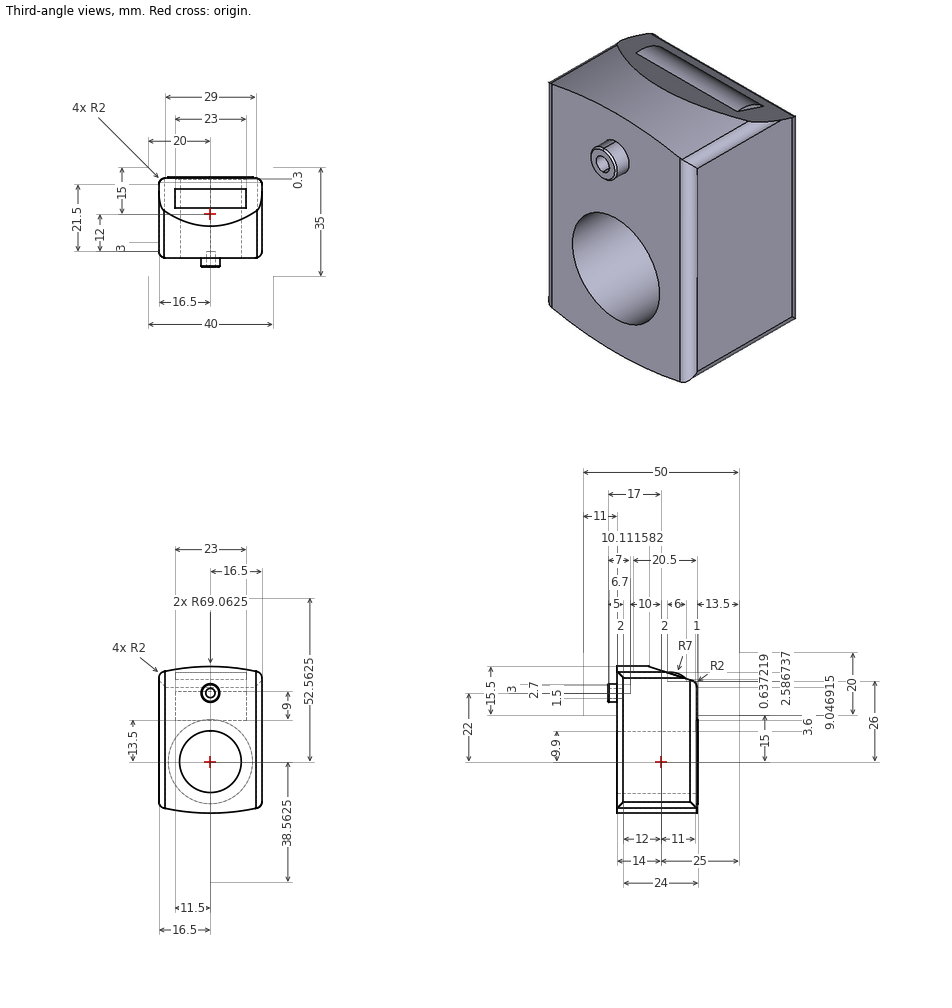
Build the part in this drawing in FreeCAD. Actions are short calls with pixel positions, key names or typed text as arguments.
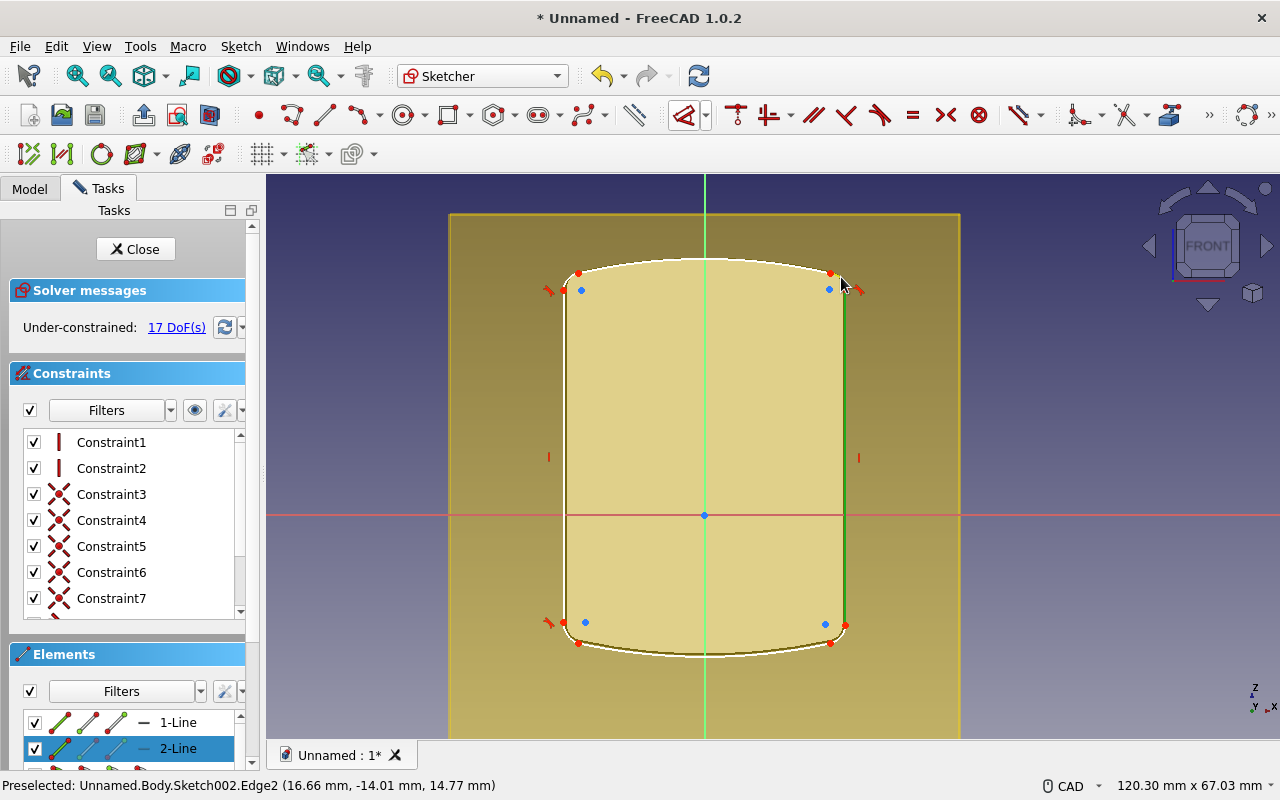
scroll(837, 640, up, 4)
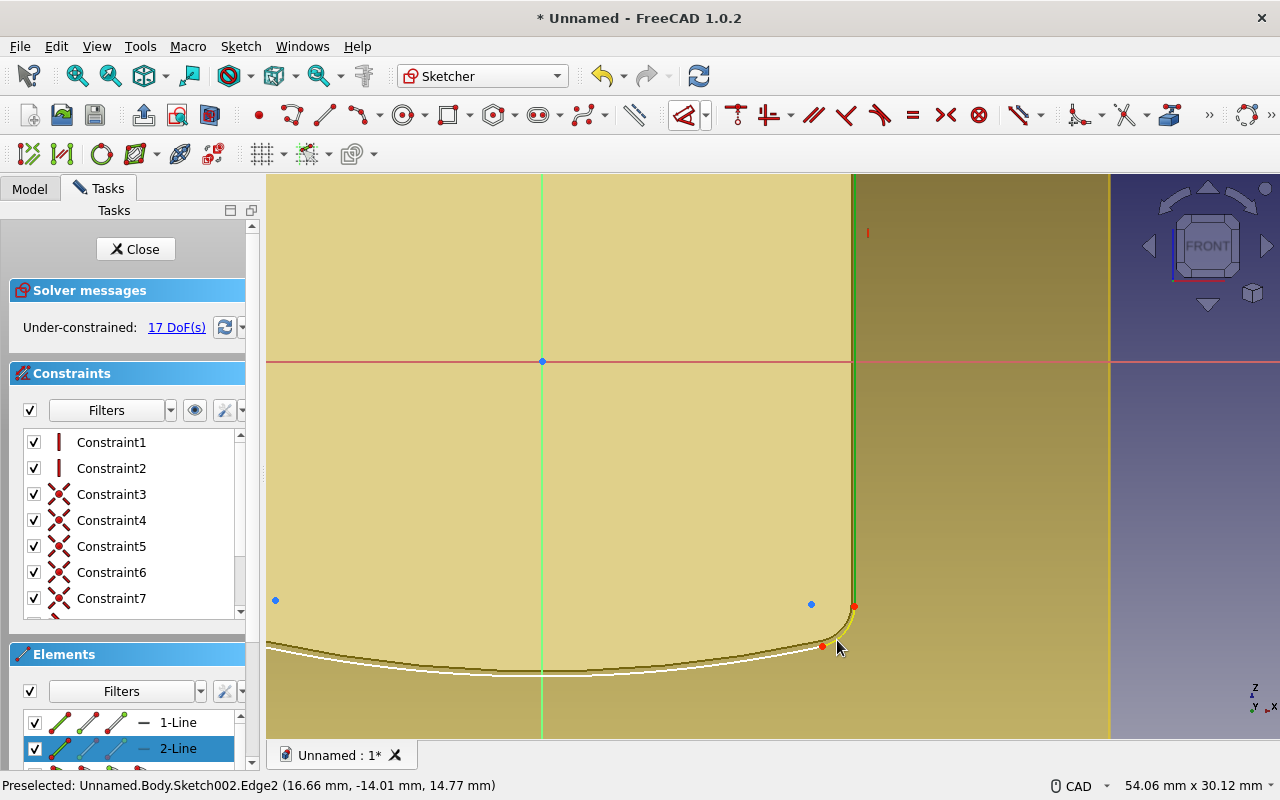
click(837, 639)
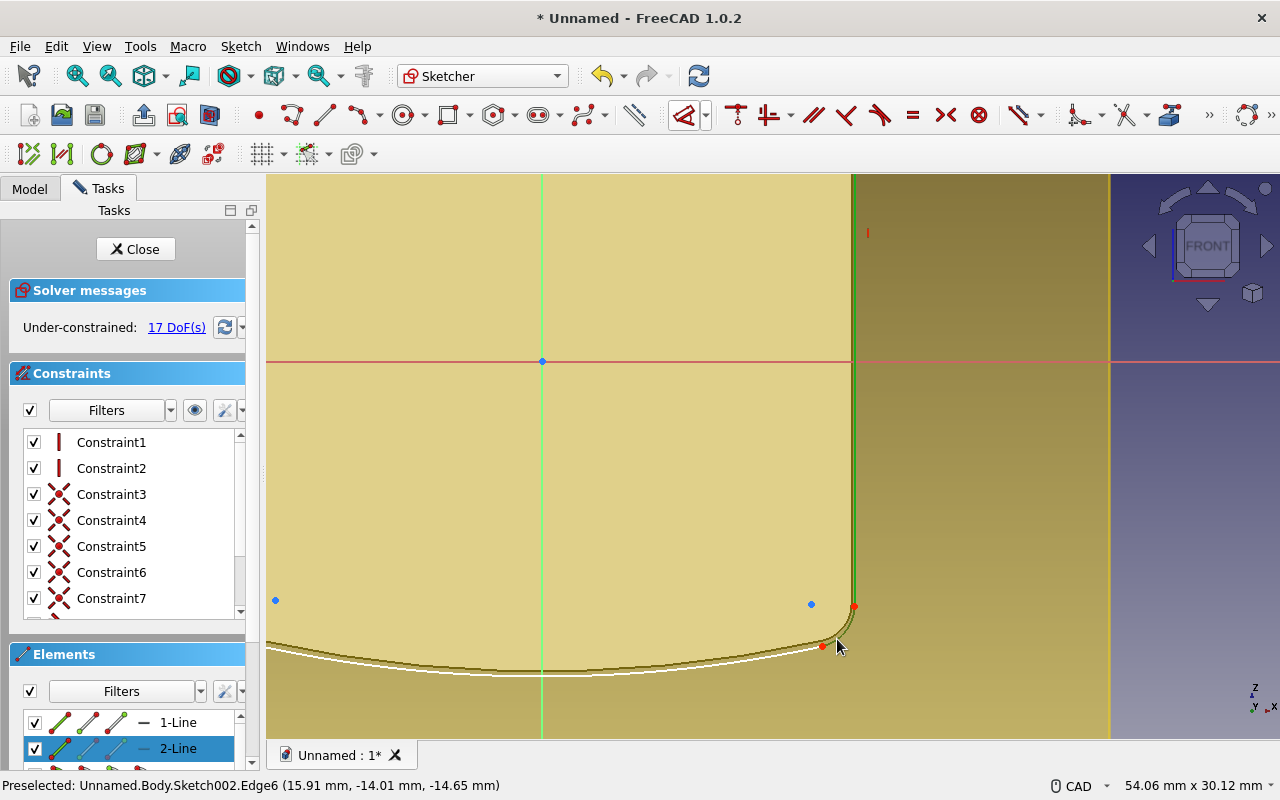
click(880, 116)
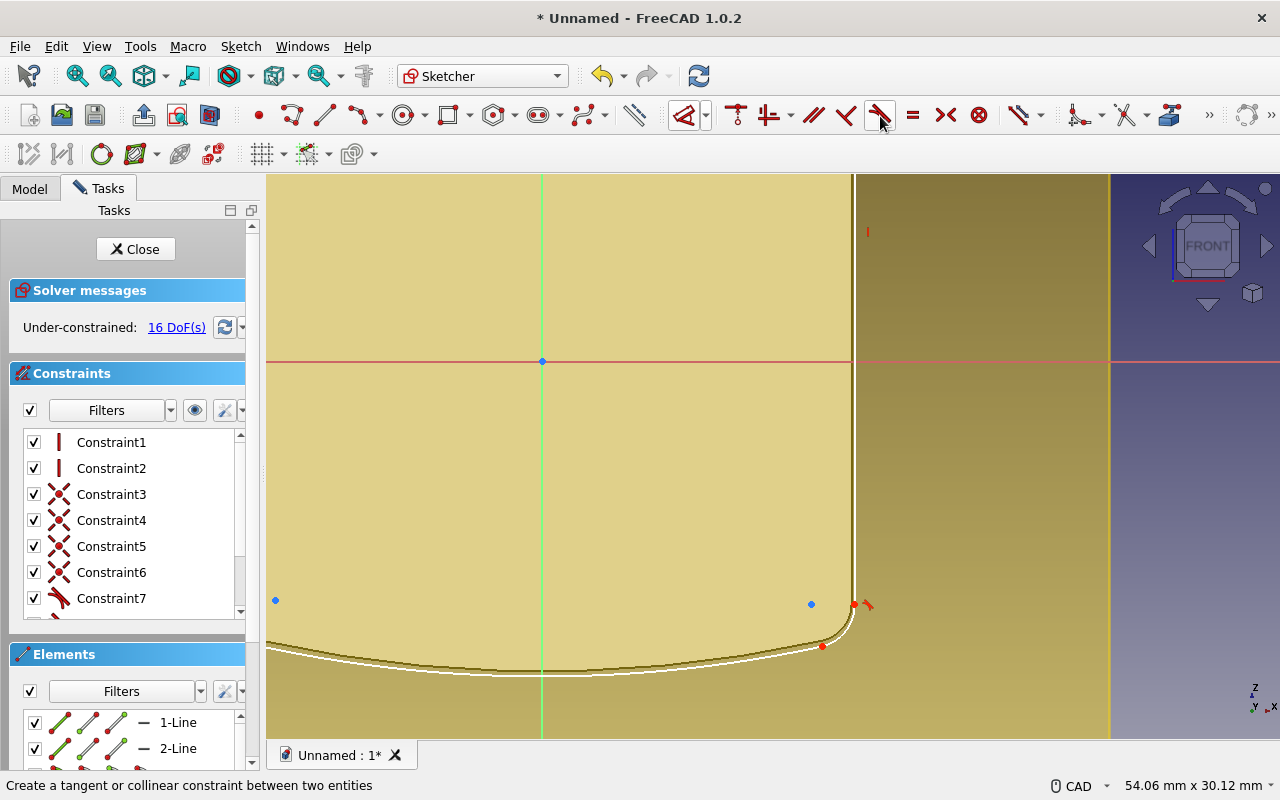
scroll(837, 641, down, 4)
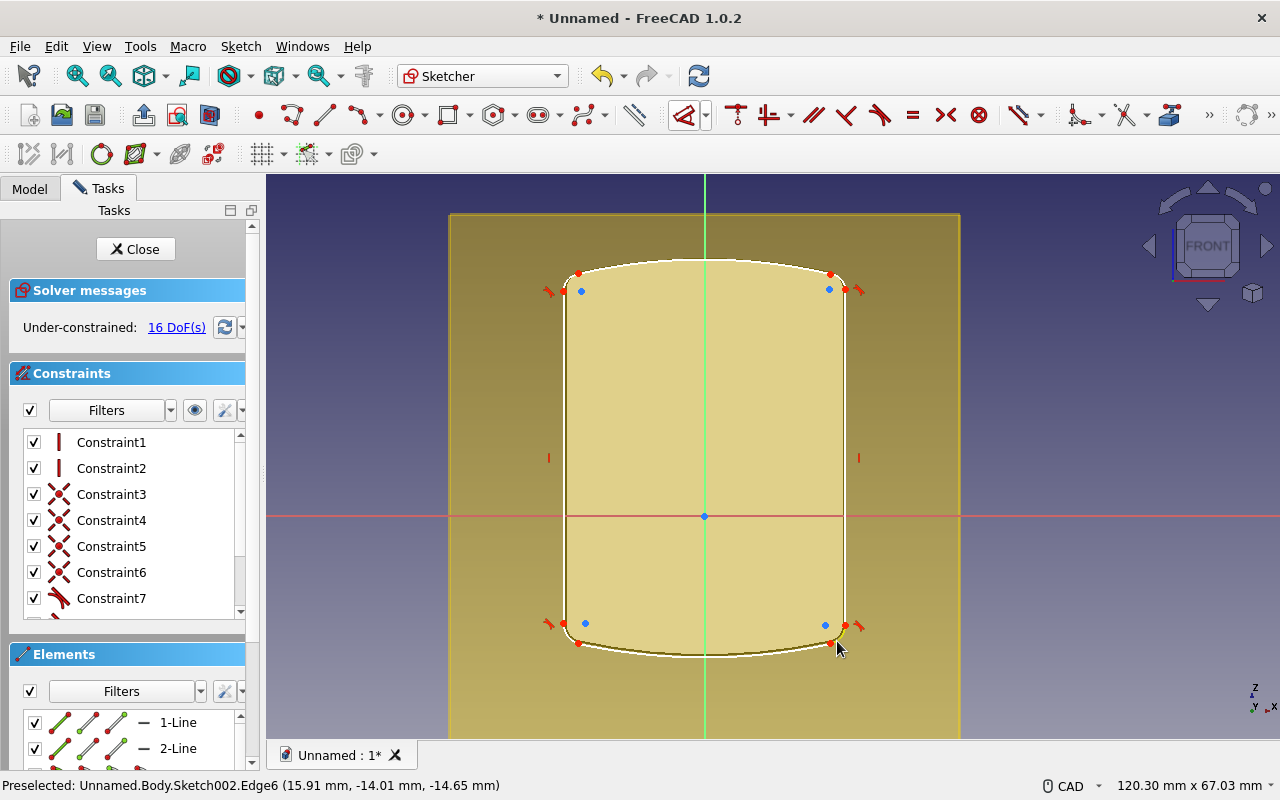
scroll(572, 277, up, 4)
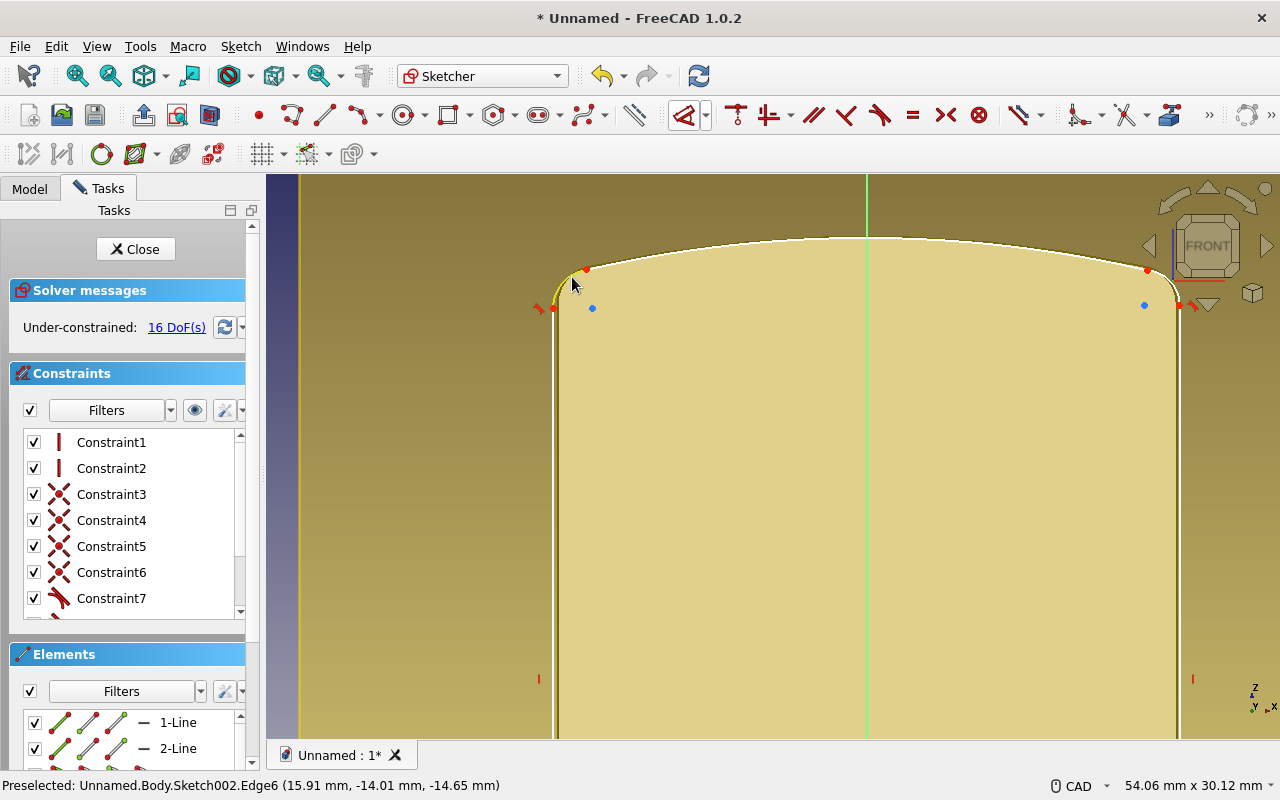
click(571, 276)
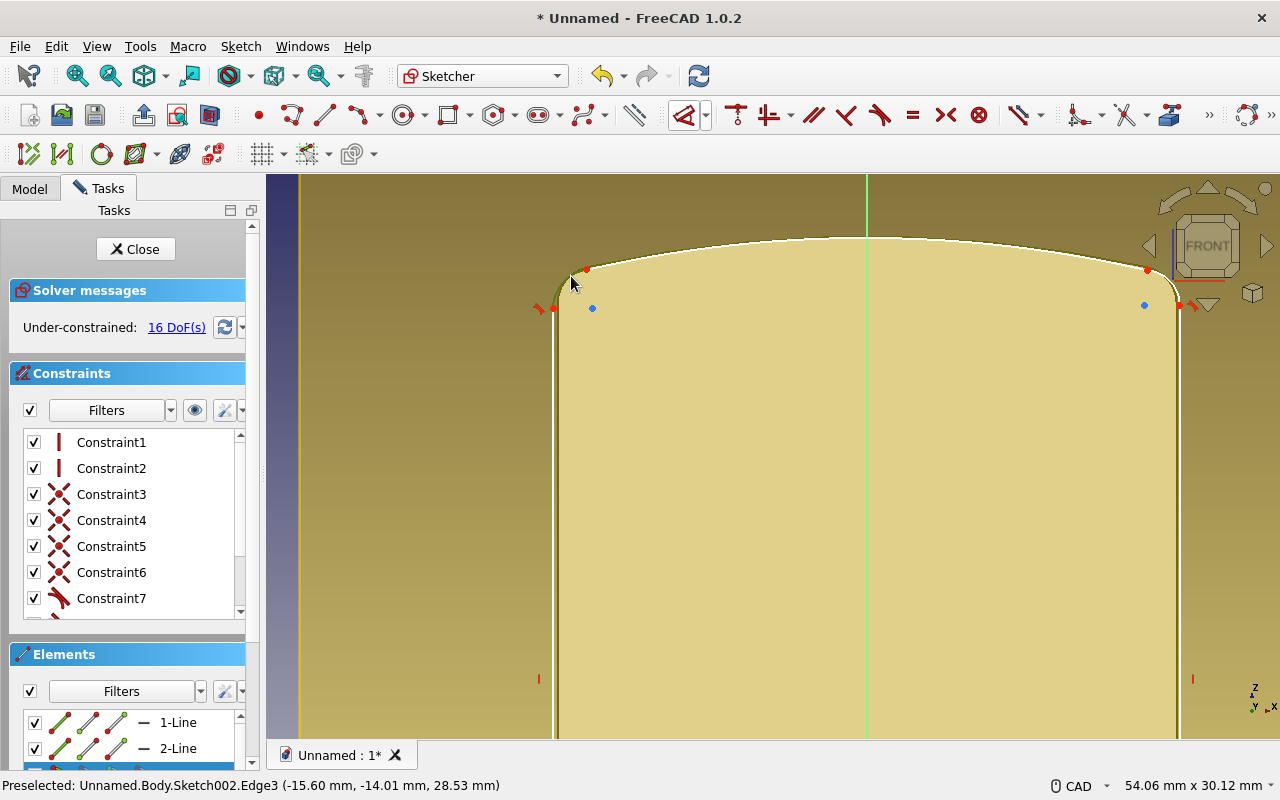
click(980, 243)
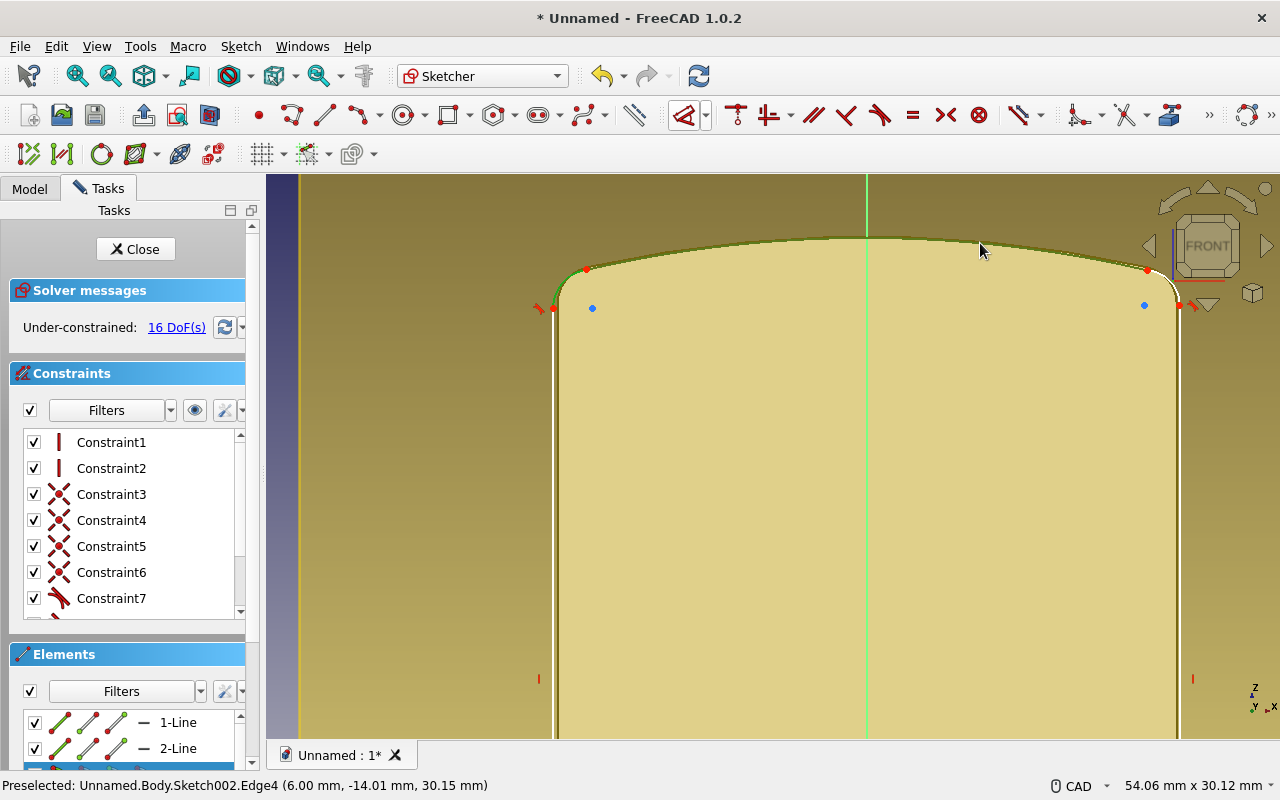
click(880, 116)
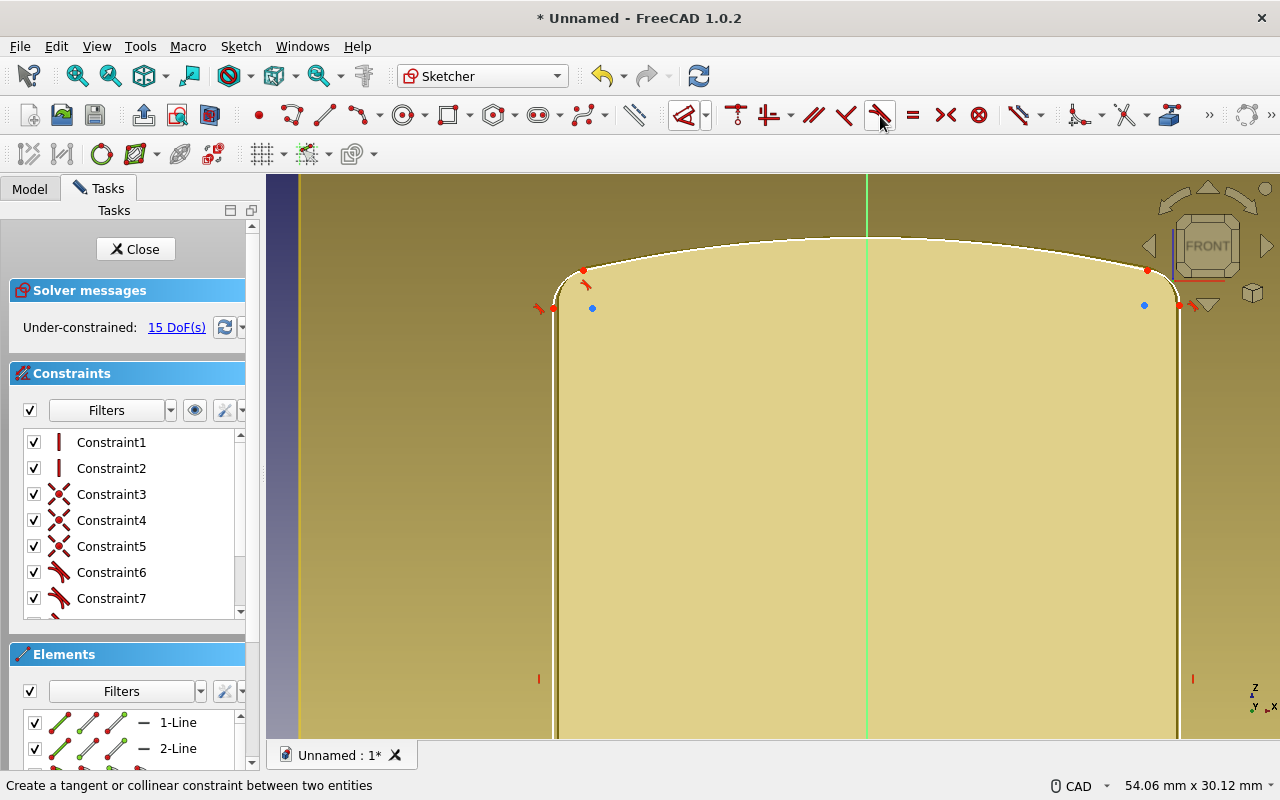
click(979, 243)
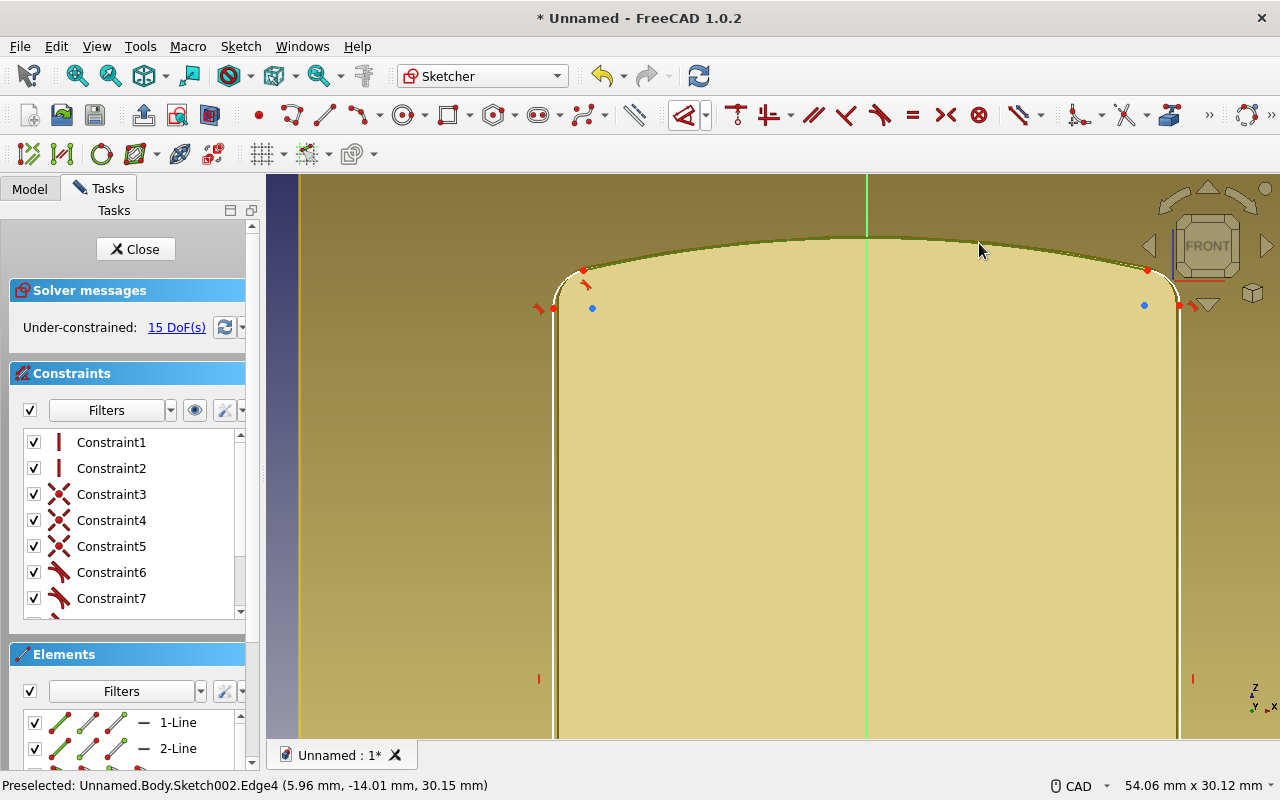
scroll(572, 276, down, 4)